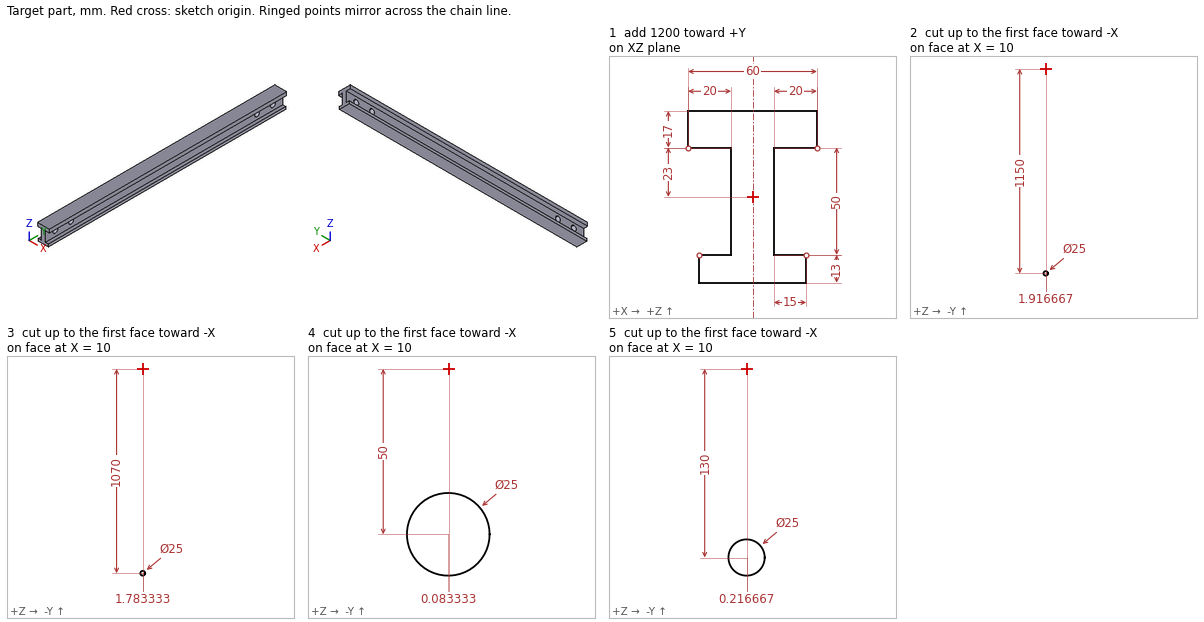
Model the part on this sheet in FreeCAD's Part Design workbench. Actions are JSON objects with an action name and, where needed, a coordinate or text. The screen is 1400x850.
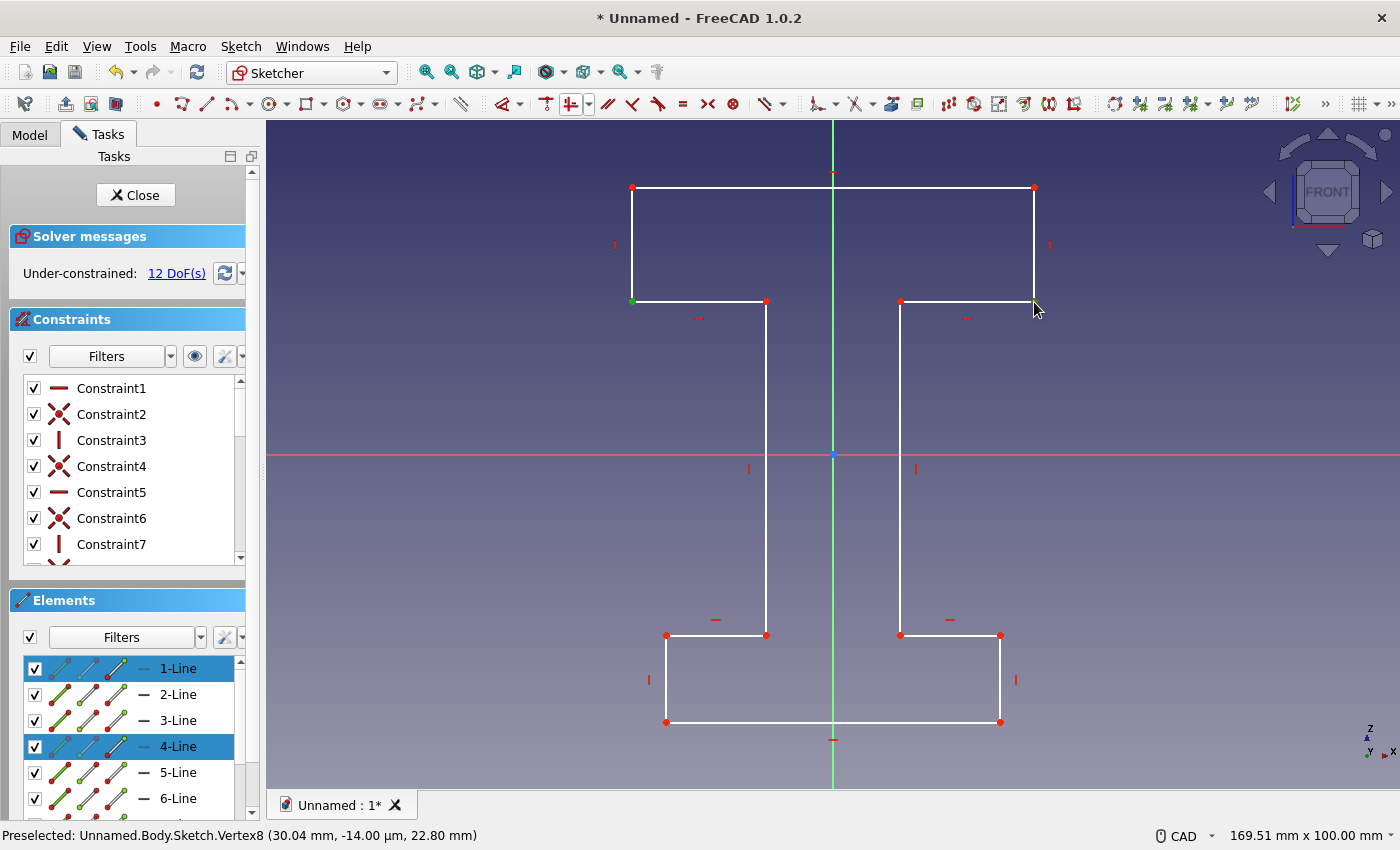
{"action": "left_click", "coordinate": [833, 673]}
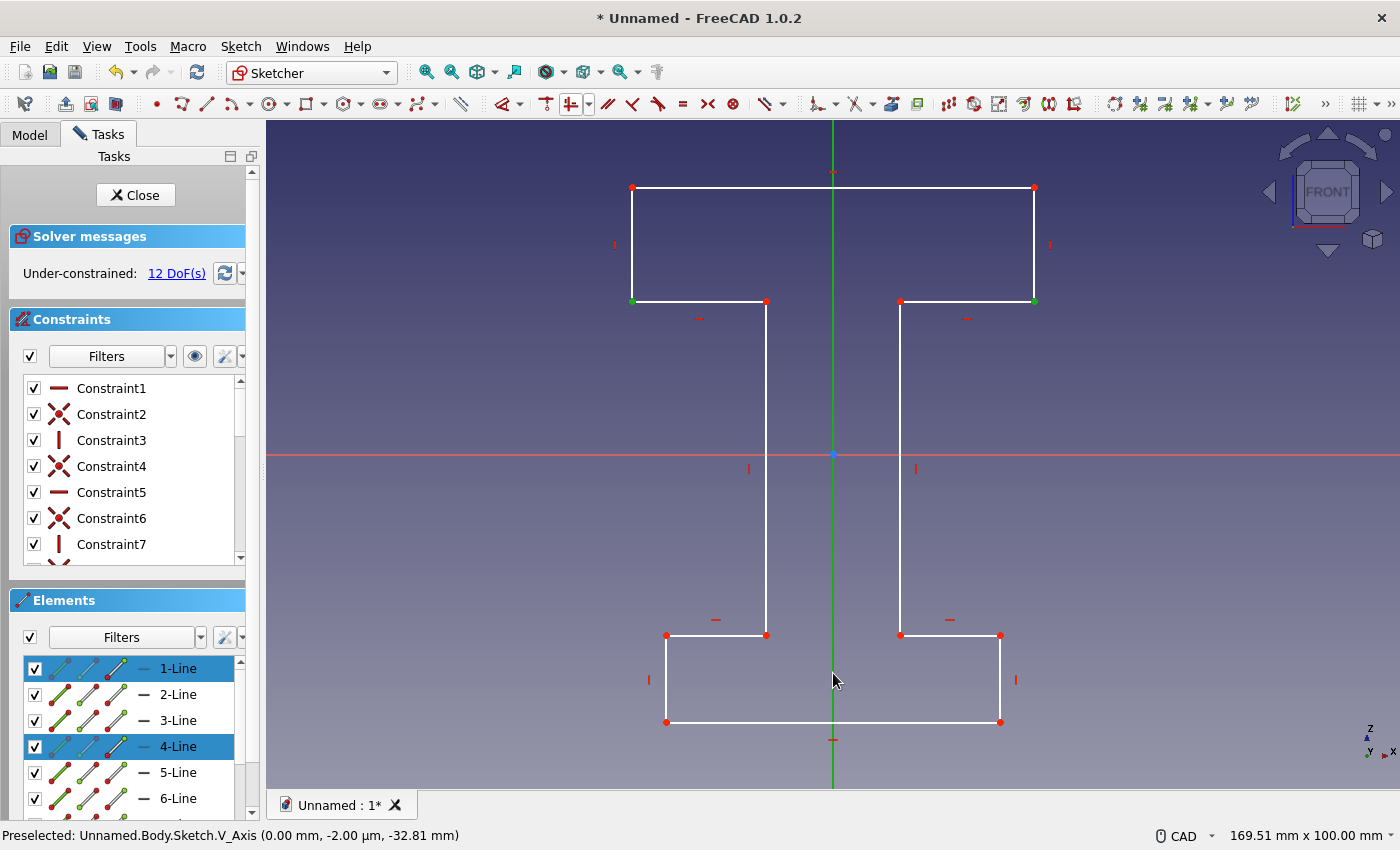
{"action": "left_click", "coordinate": [708, 104]}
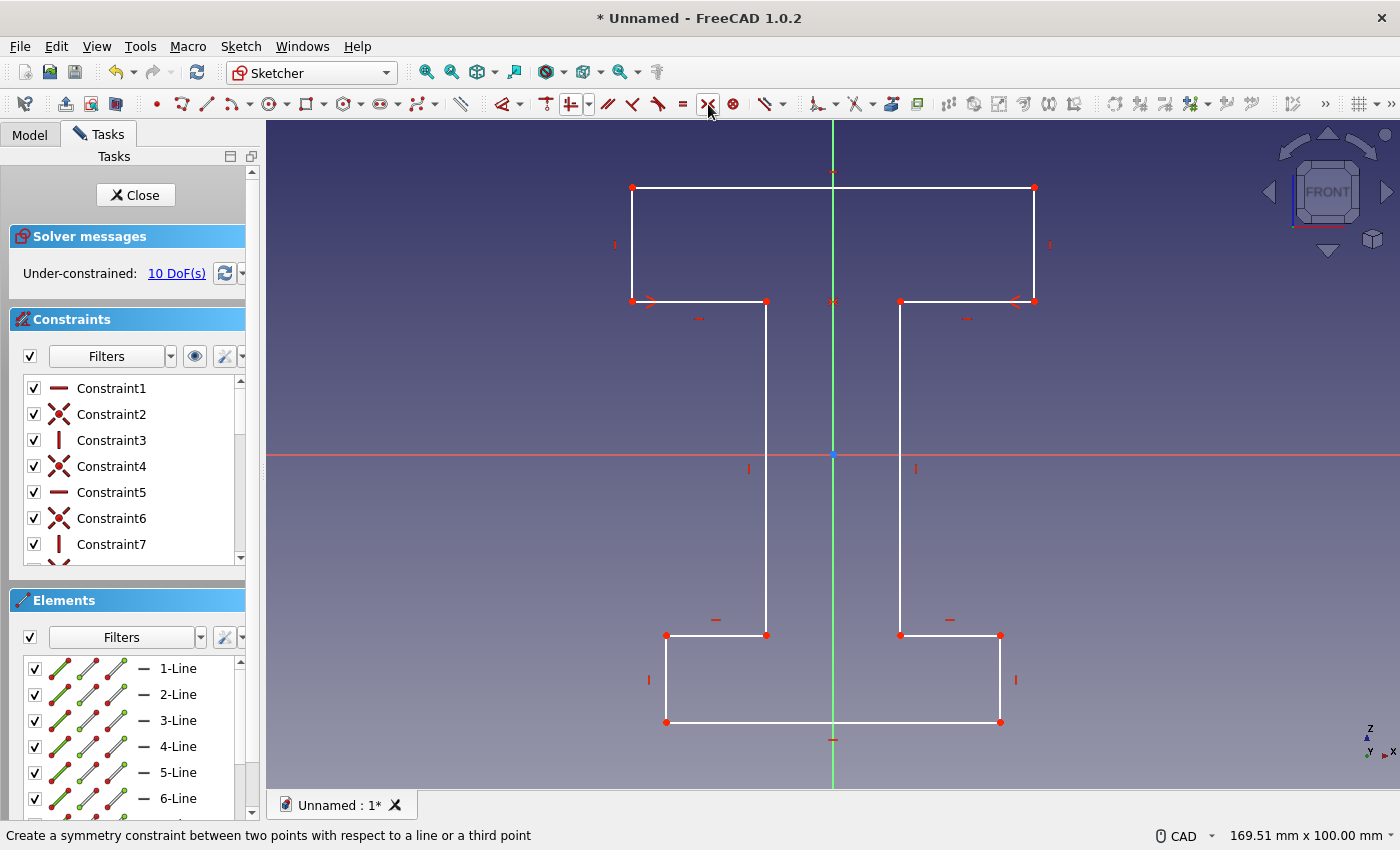
{"action": "left_click", "coordinate": [1000, 636]}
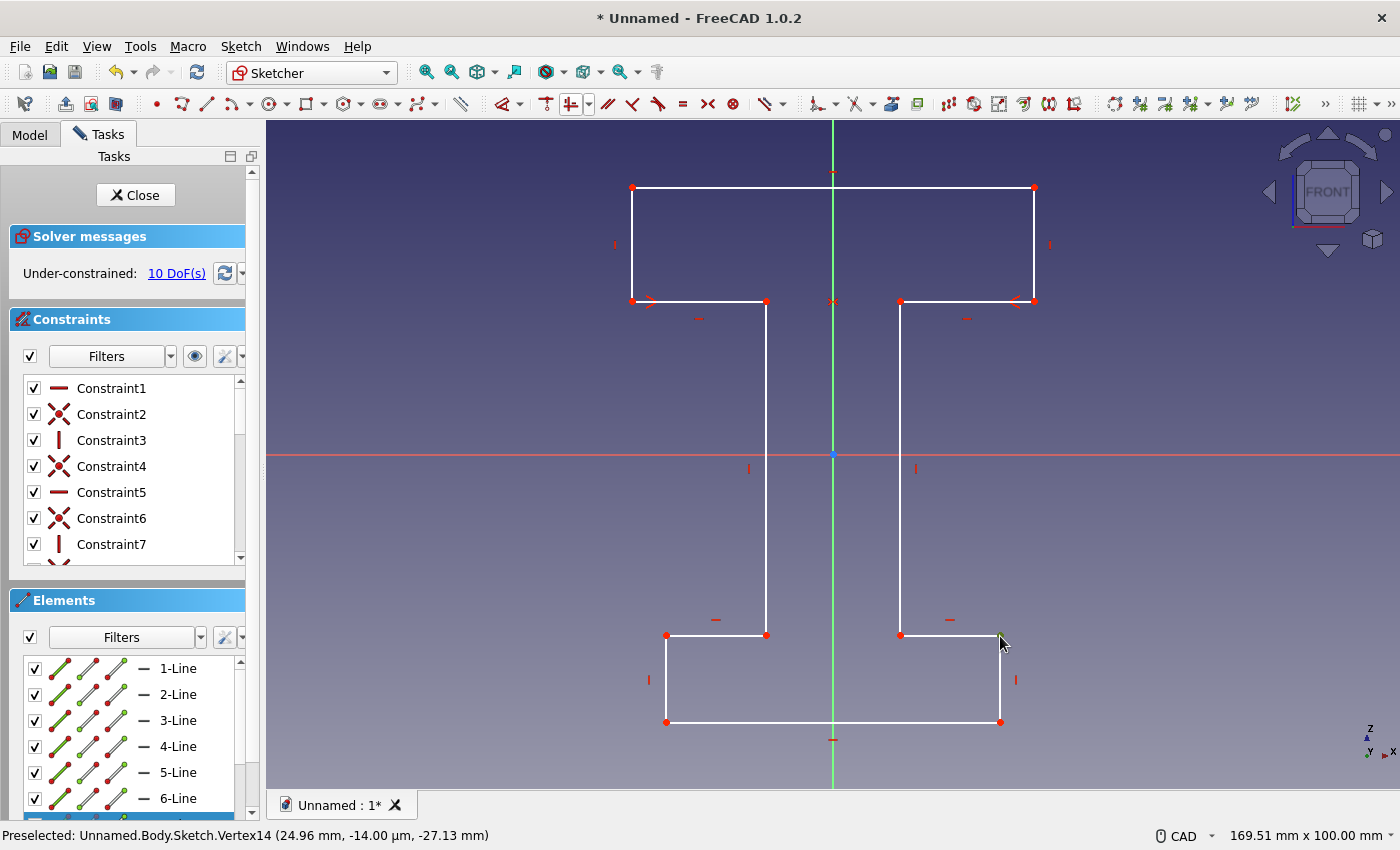
{"action": "left_click", "coordinate": [666, 636]}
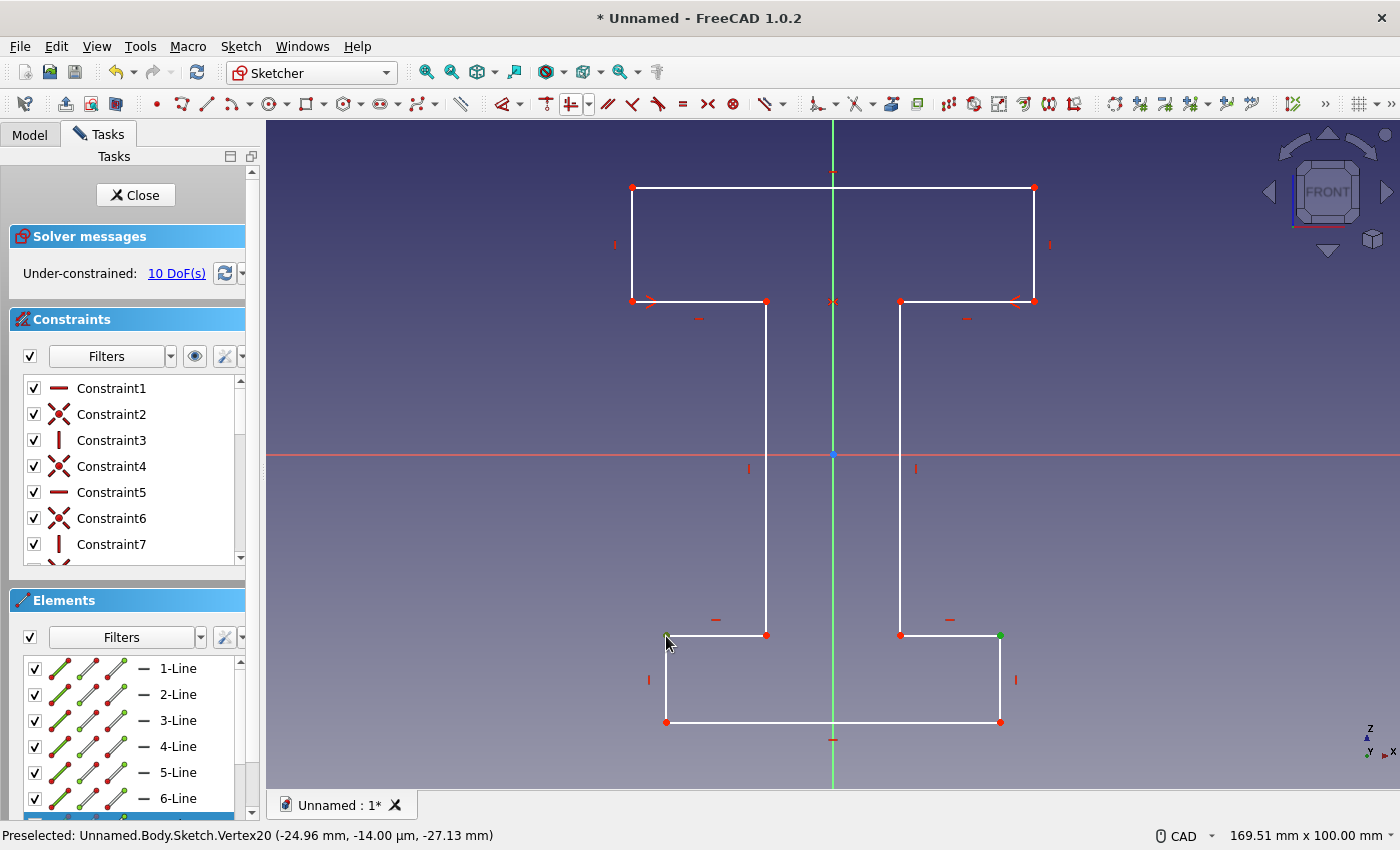
{"action": "left_click", "coordinate": [833, 673]}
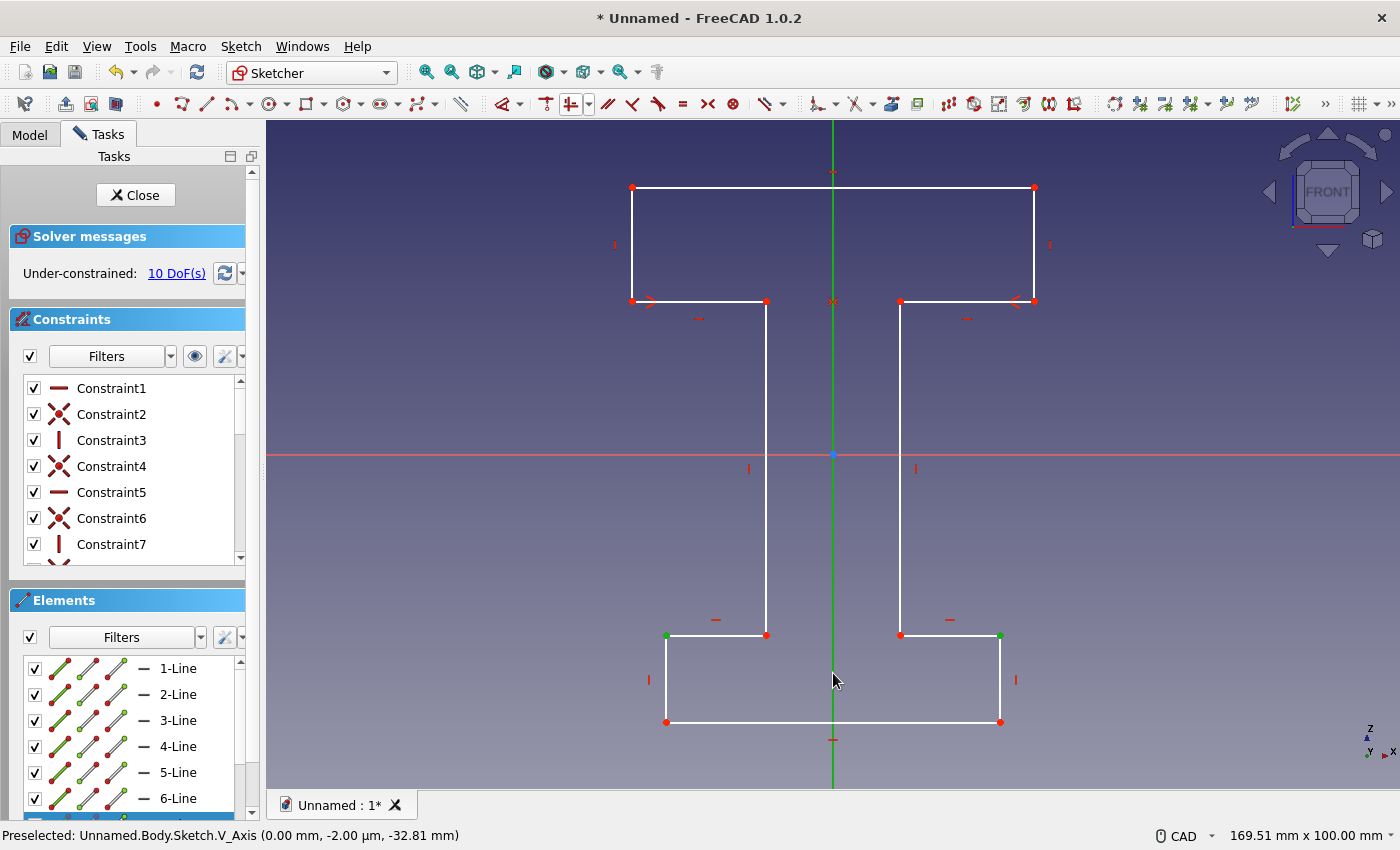
{"action": "key", "text": "s"}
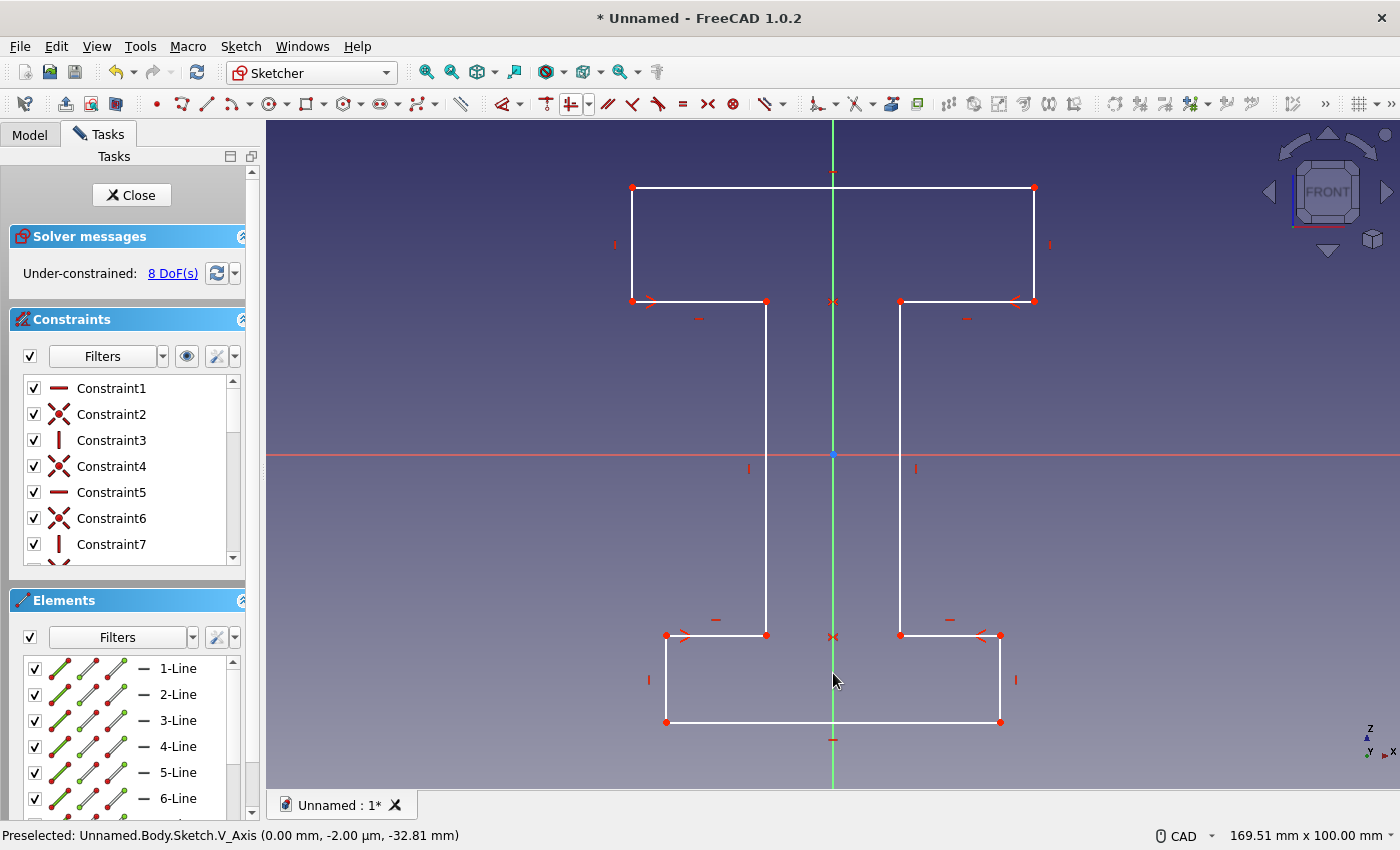
{"action": "left_click", "coordinate": [726, 302]}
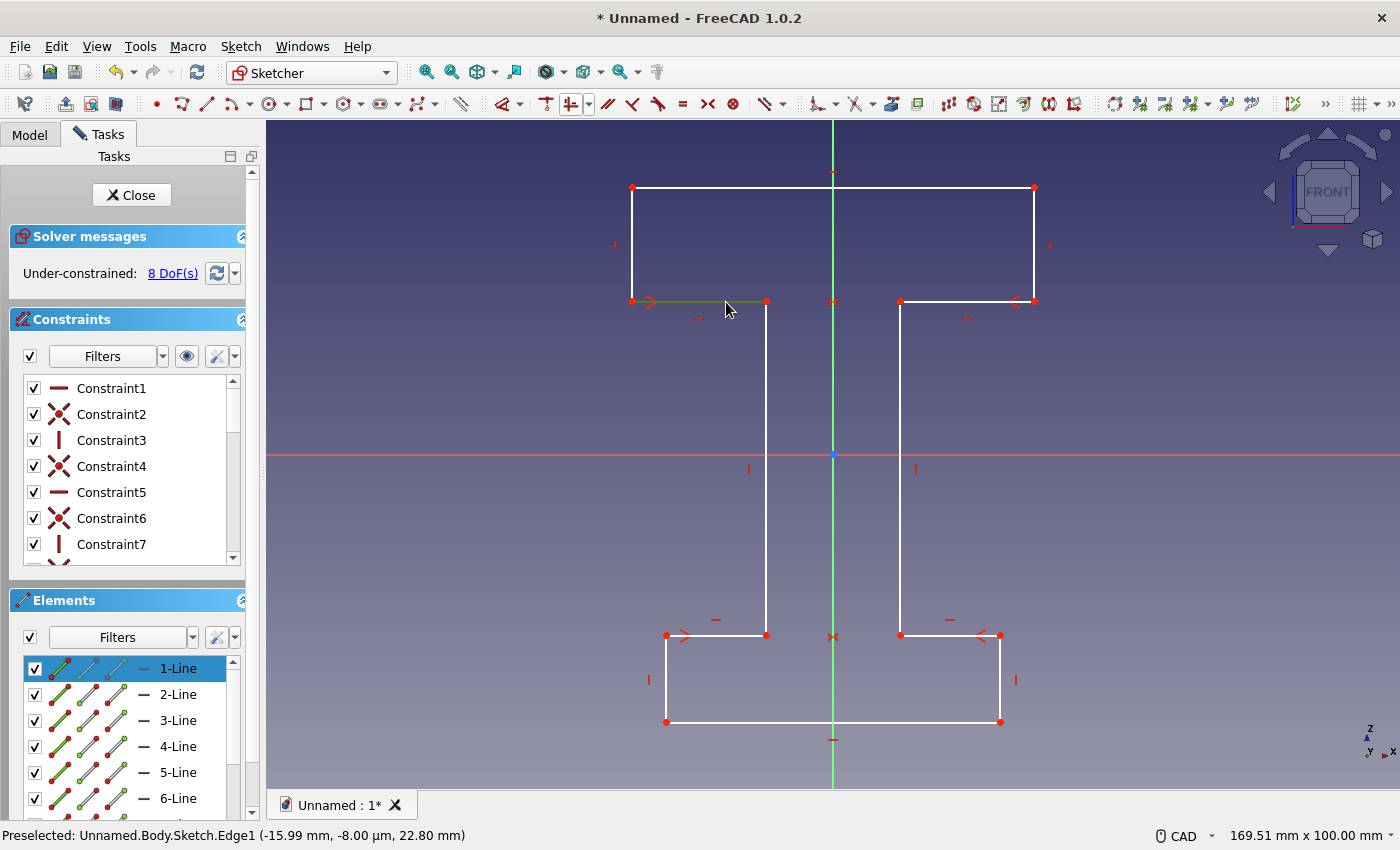
{"action": "left_click", "coordinate": [520, 104]}